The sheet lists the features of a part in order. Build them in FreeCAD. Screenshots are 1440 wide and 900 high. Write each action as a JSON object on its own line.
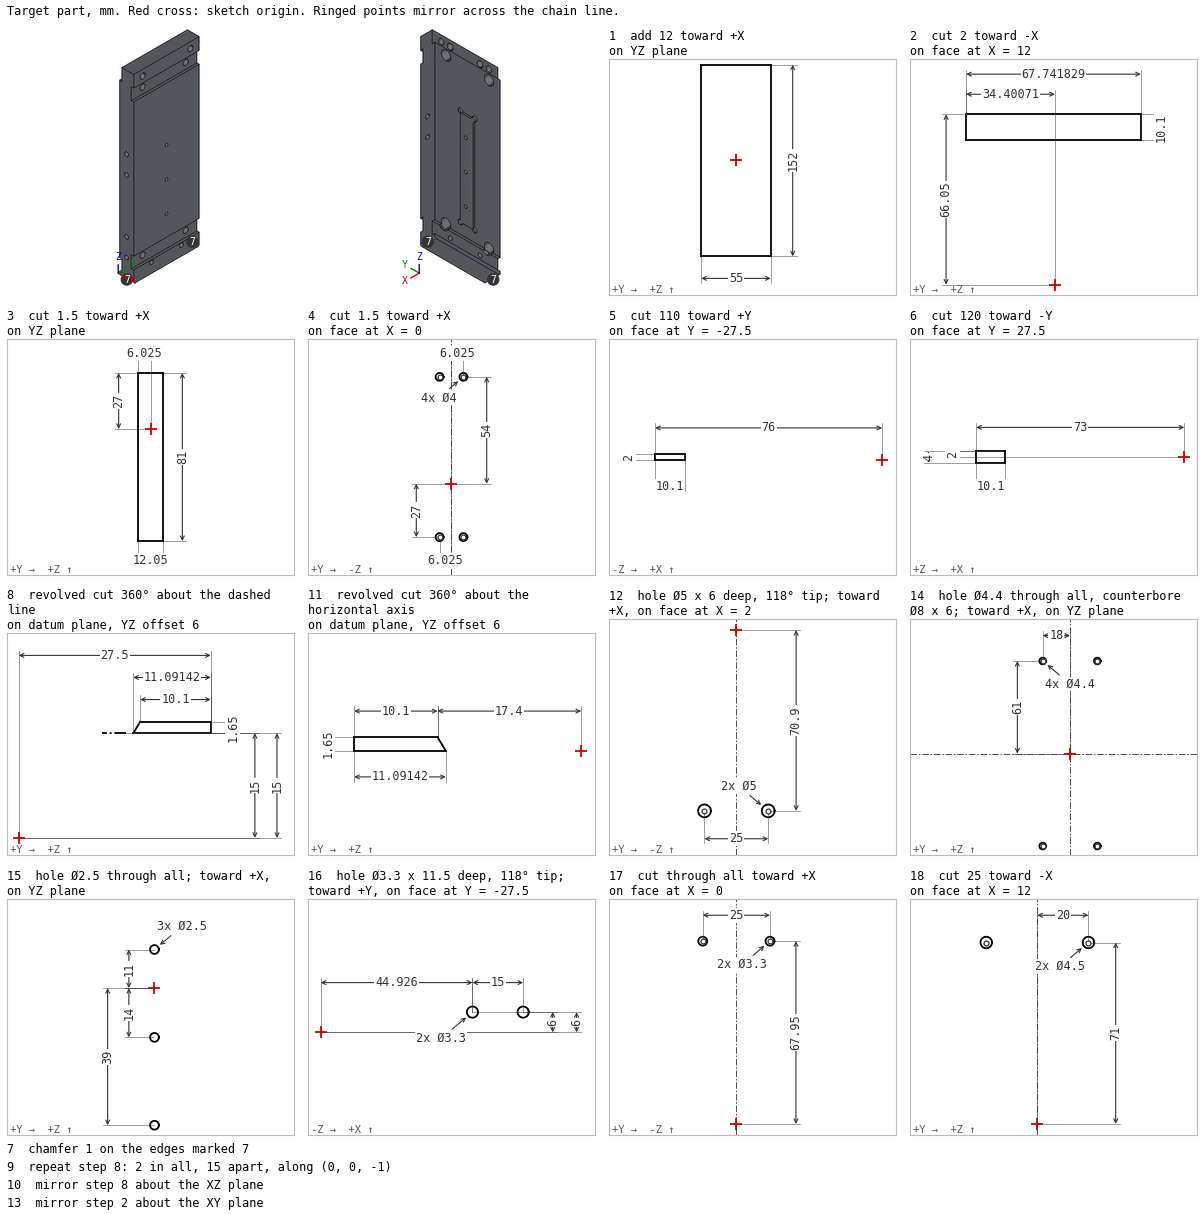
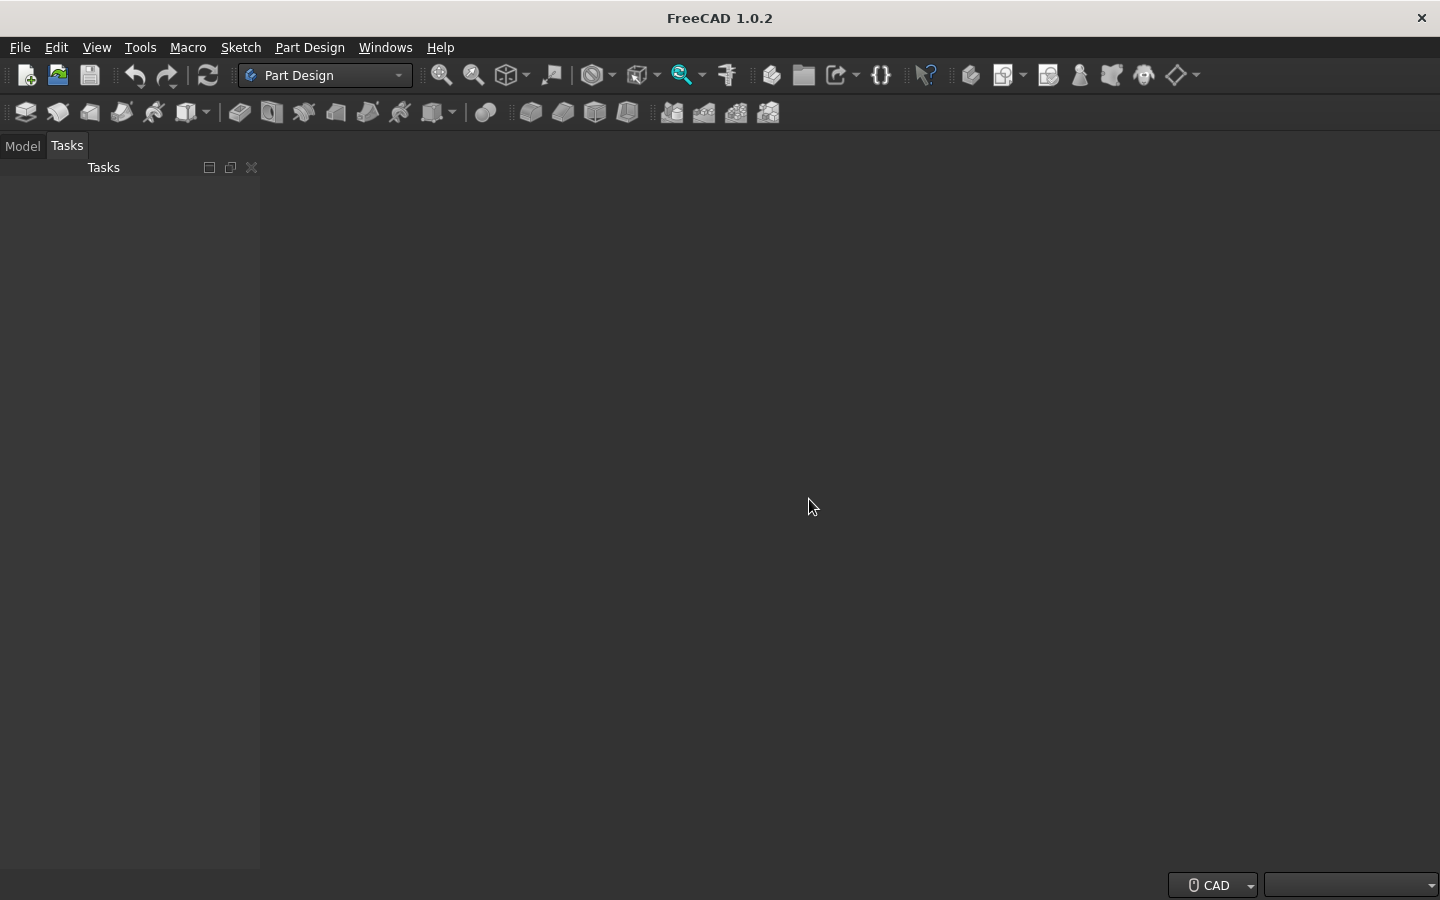
{"action": "left_click", "coordinate": [26, 76]}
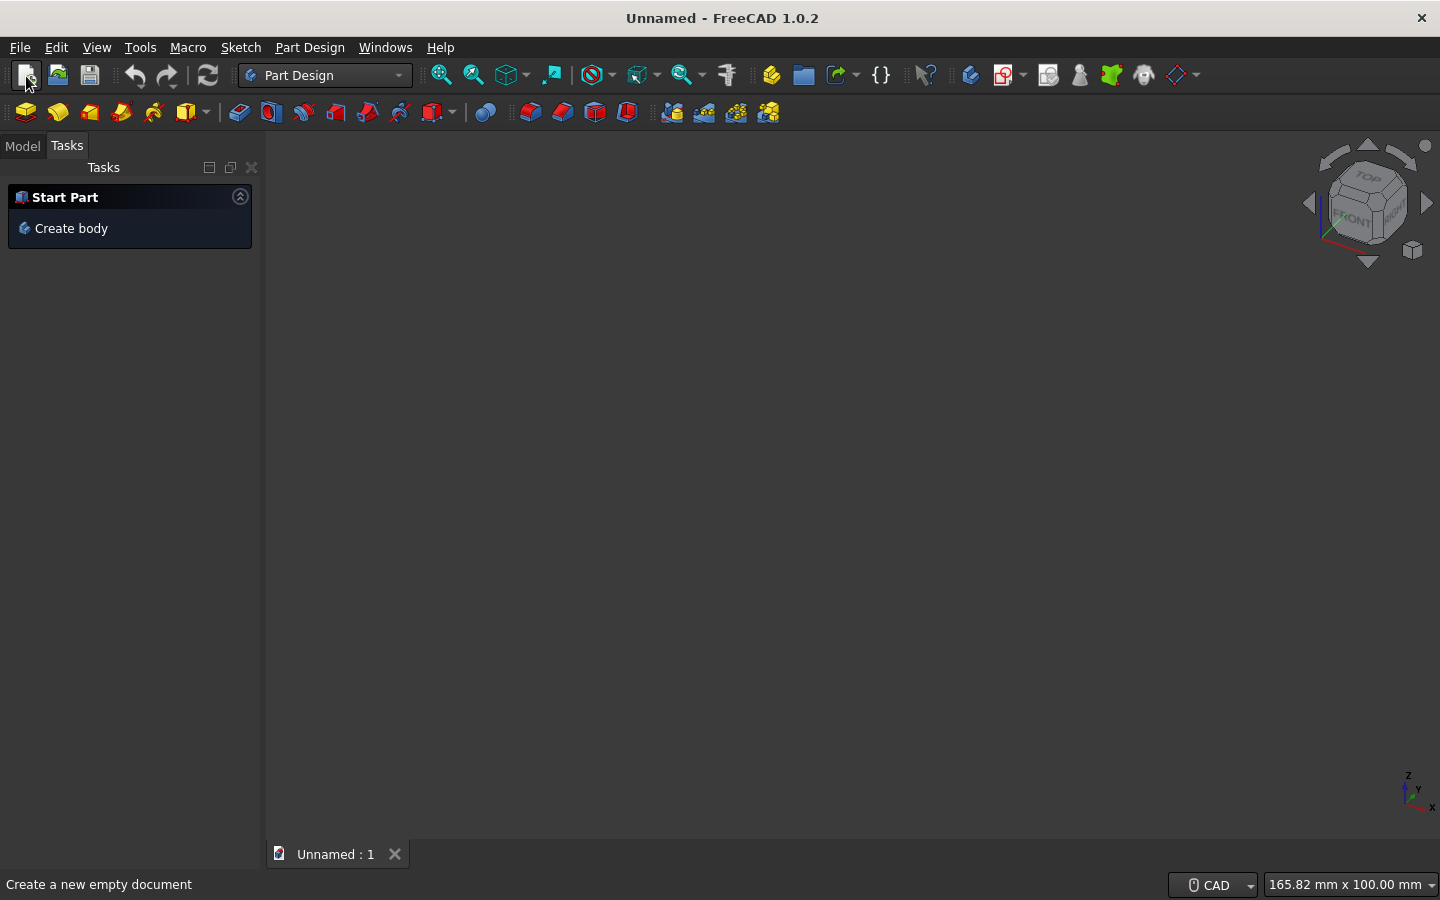
{"action": "left_click", "coordinate": [1004, 76]}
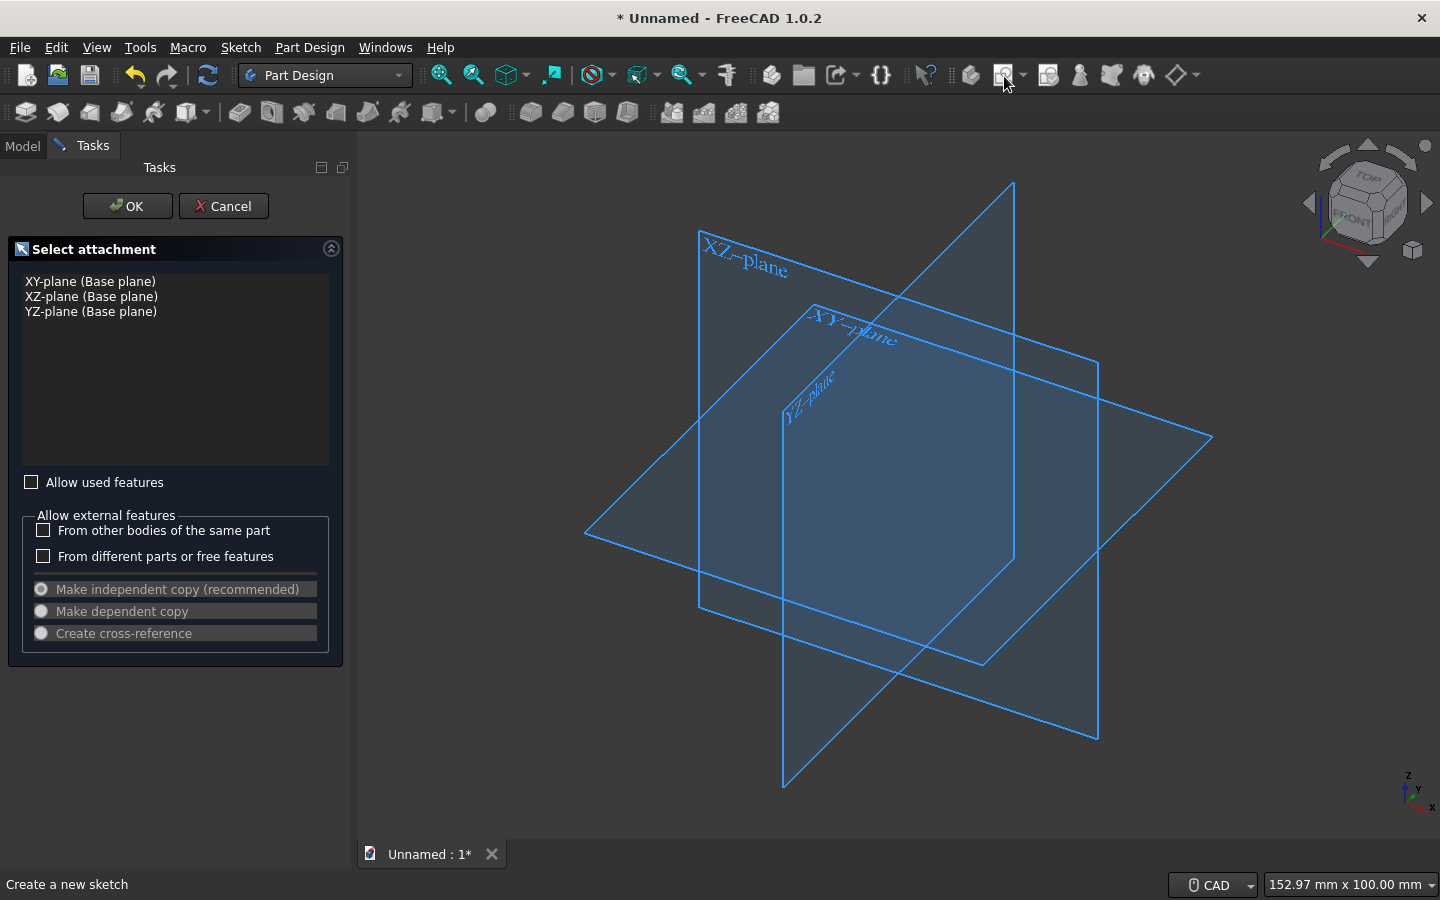
{"action": "left_click", "coordinate": [82, 312]}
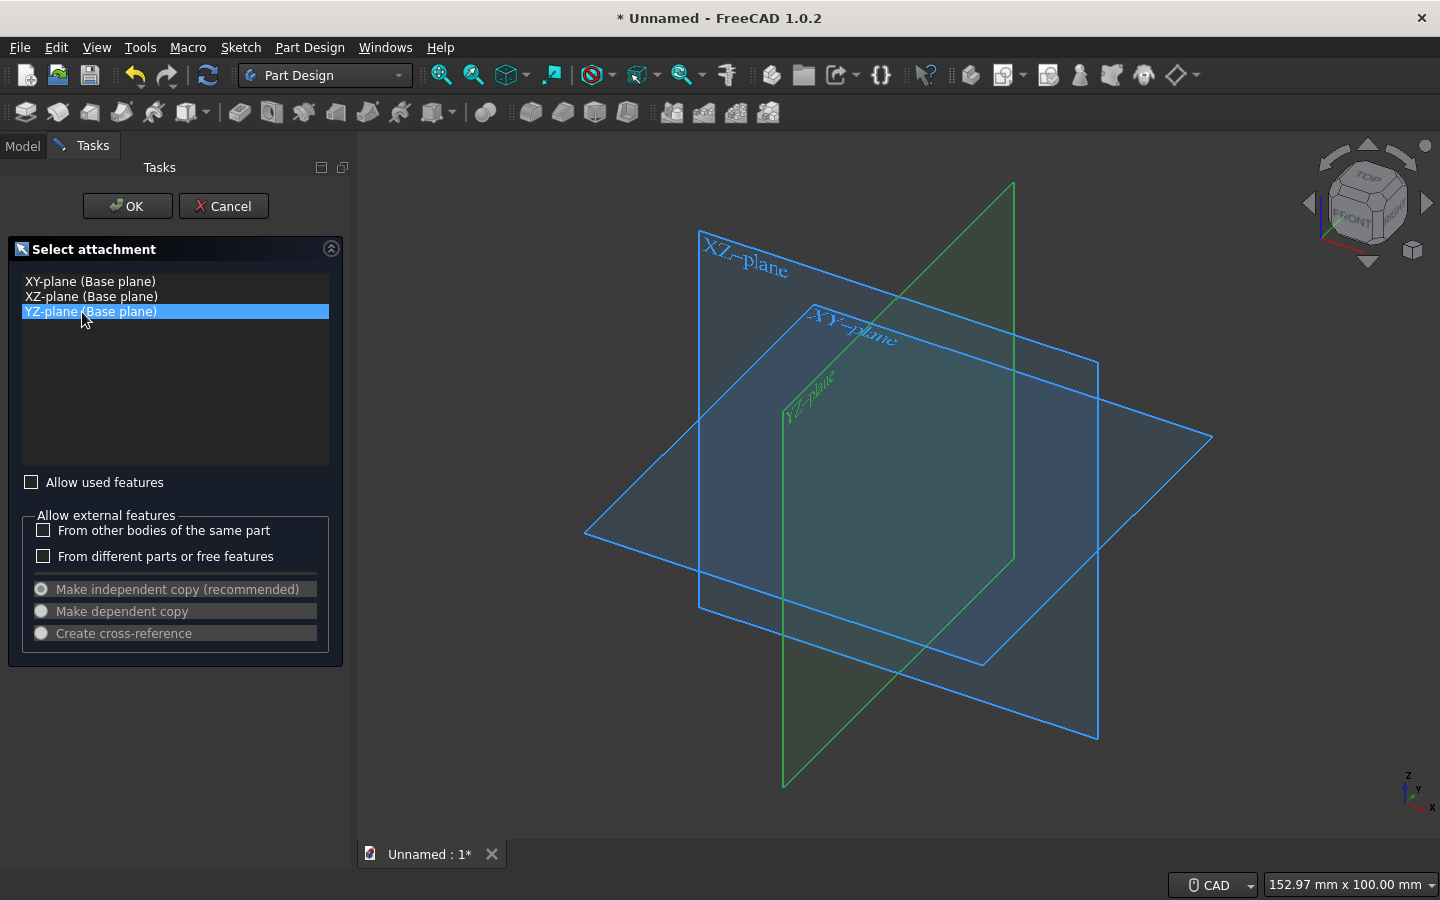
{"action": "left_click", "coordinate": [128, 206]}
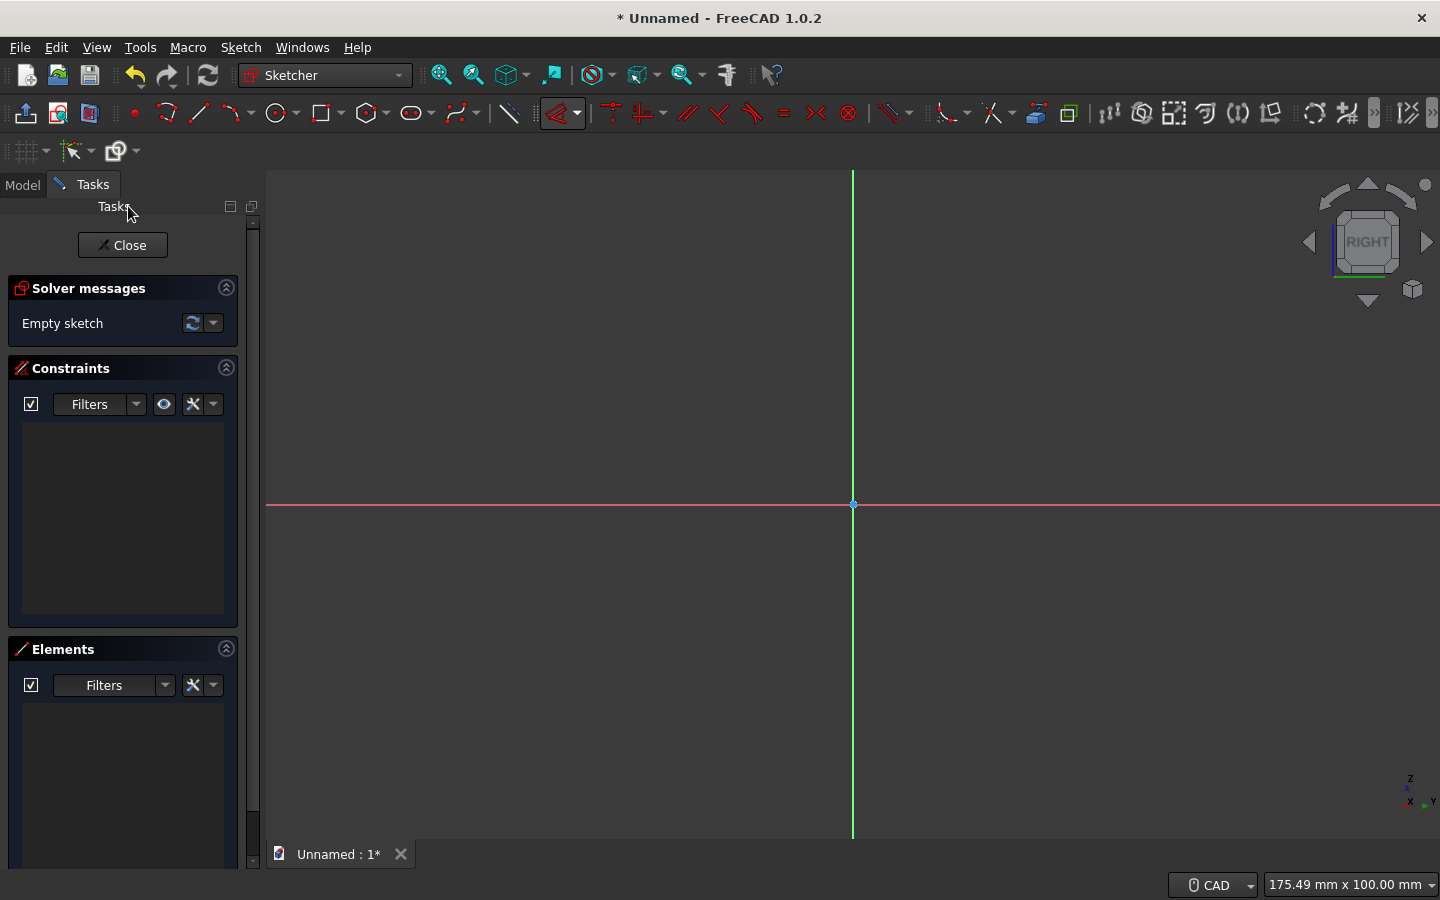
{"action": "scroll", "coordinate": [729, 505], "scroll_direction": "down", "scroll_amount": 4}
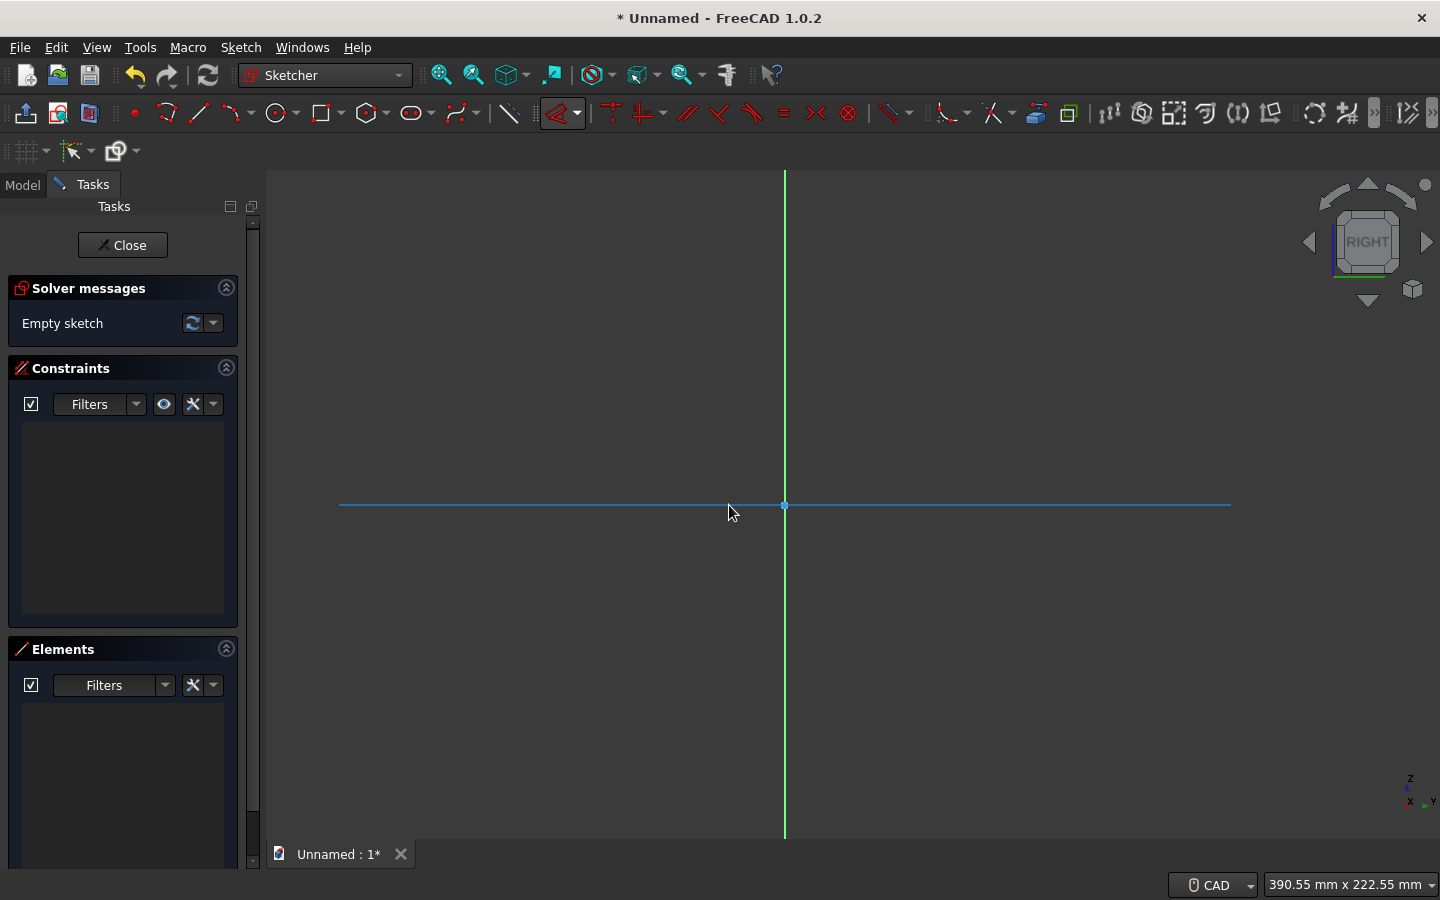
{"action": "left_click", "coordinate": [344, 114]}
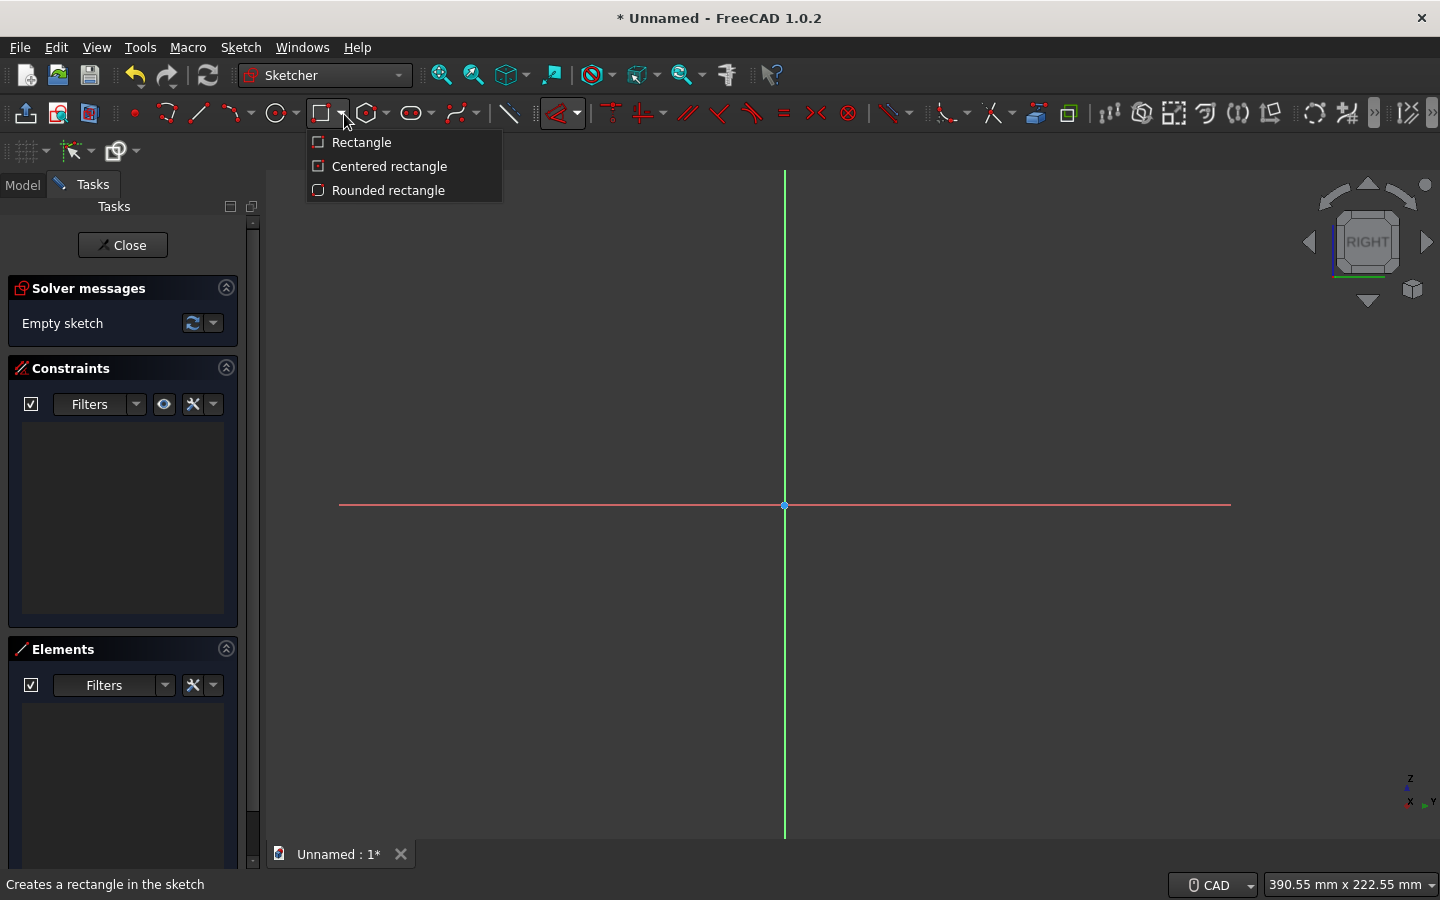
{"action": "left_click", "coordinate": [404, 166]}